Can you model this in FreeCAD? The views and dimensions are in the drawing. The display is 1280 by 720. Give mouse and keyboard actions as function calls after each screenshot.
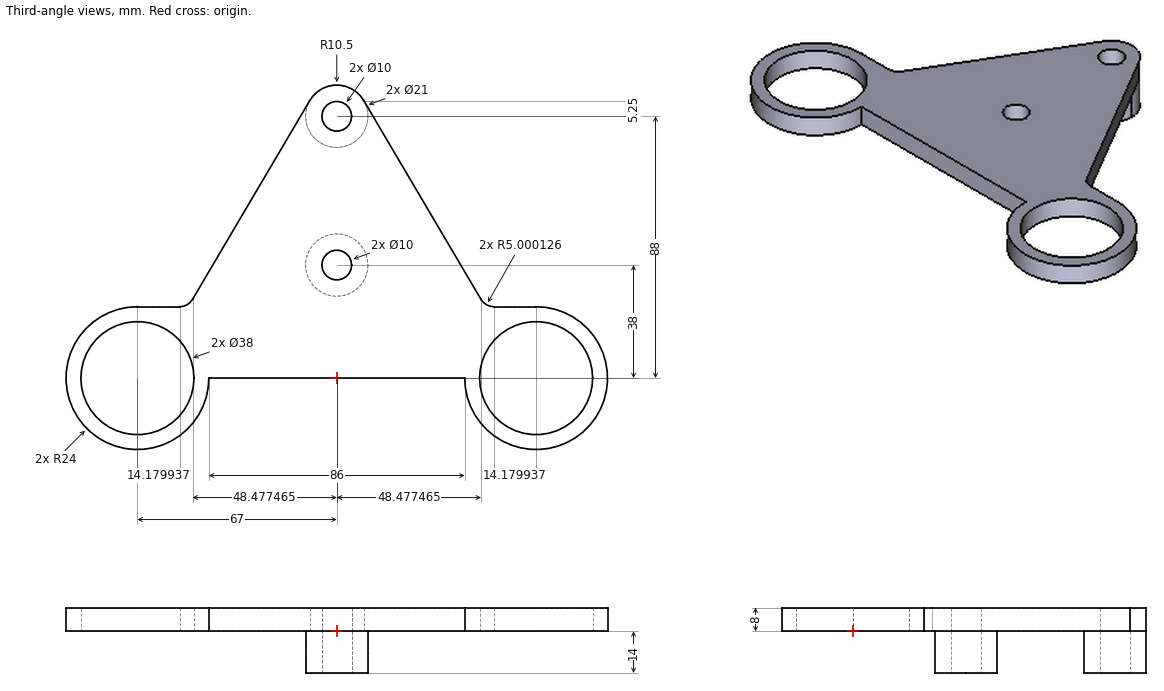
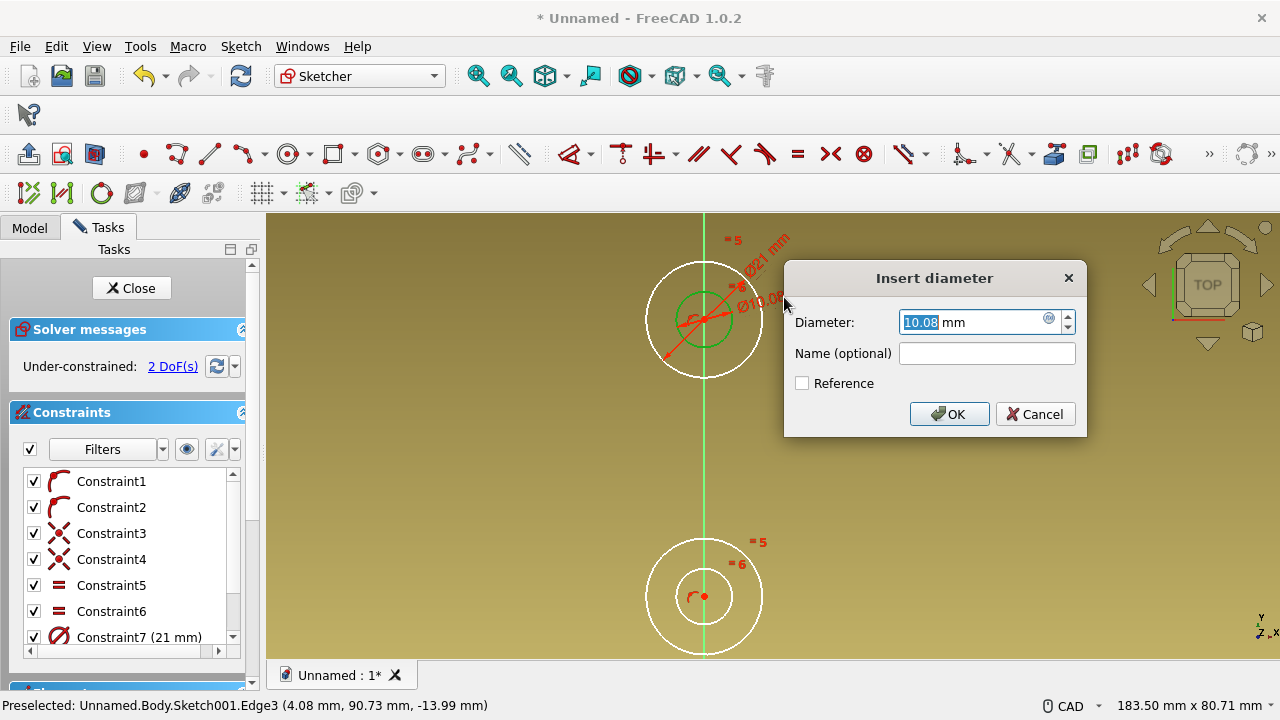
text(10)
key(Return)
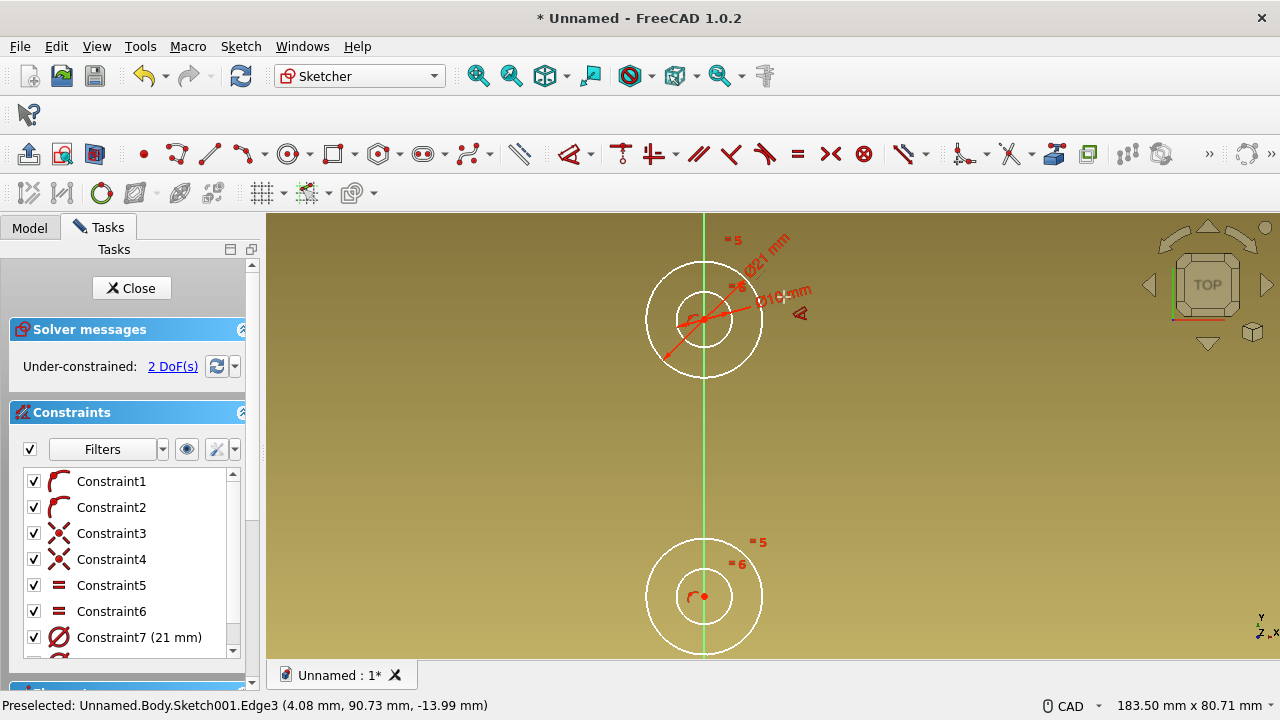
click(704, 320)
click(738, 475)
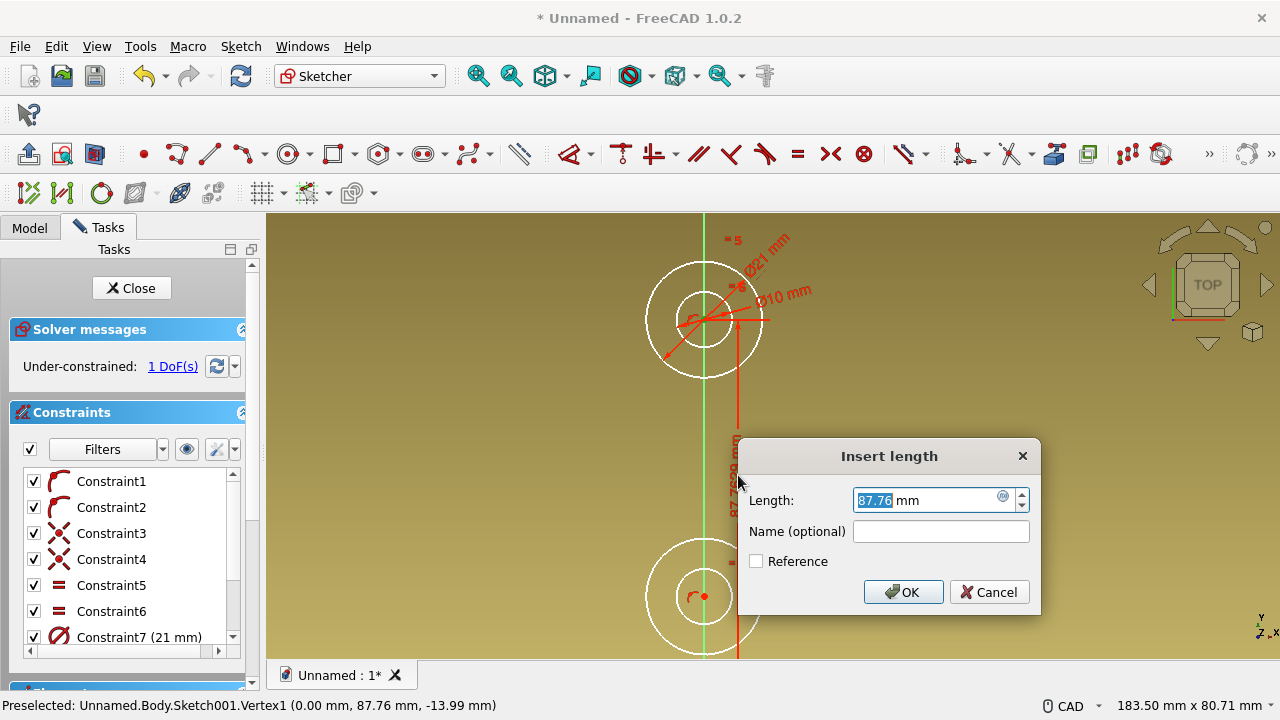
text(88)
key(Return)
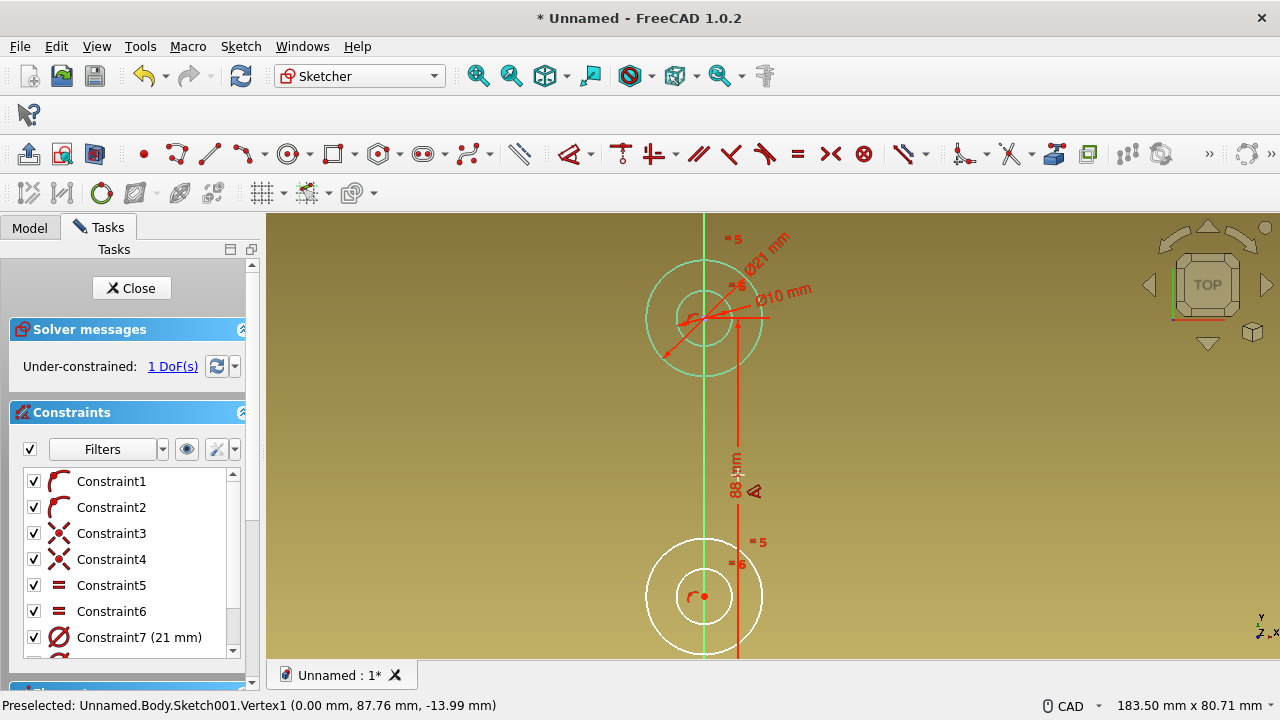
click(704, 597)
click(738, 622)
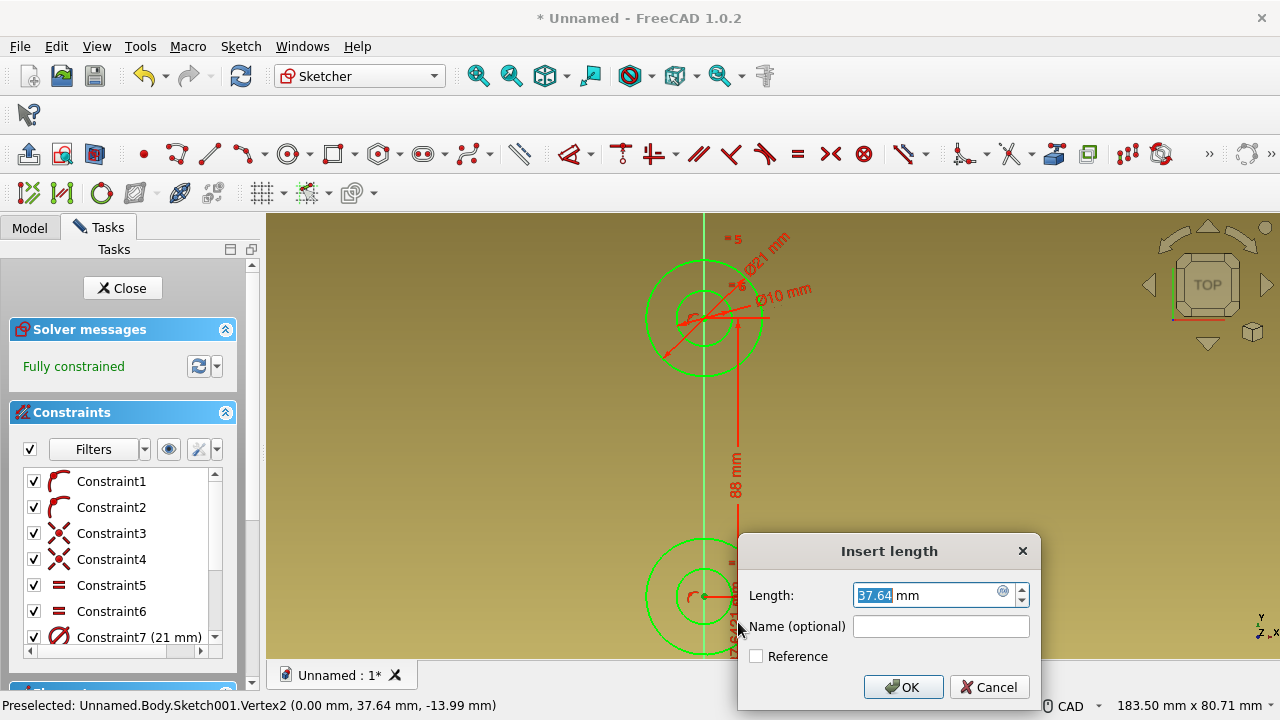
text(38)
key(Return)
key(Escape)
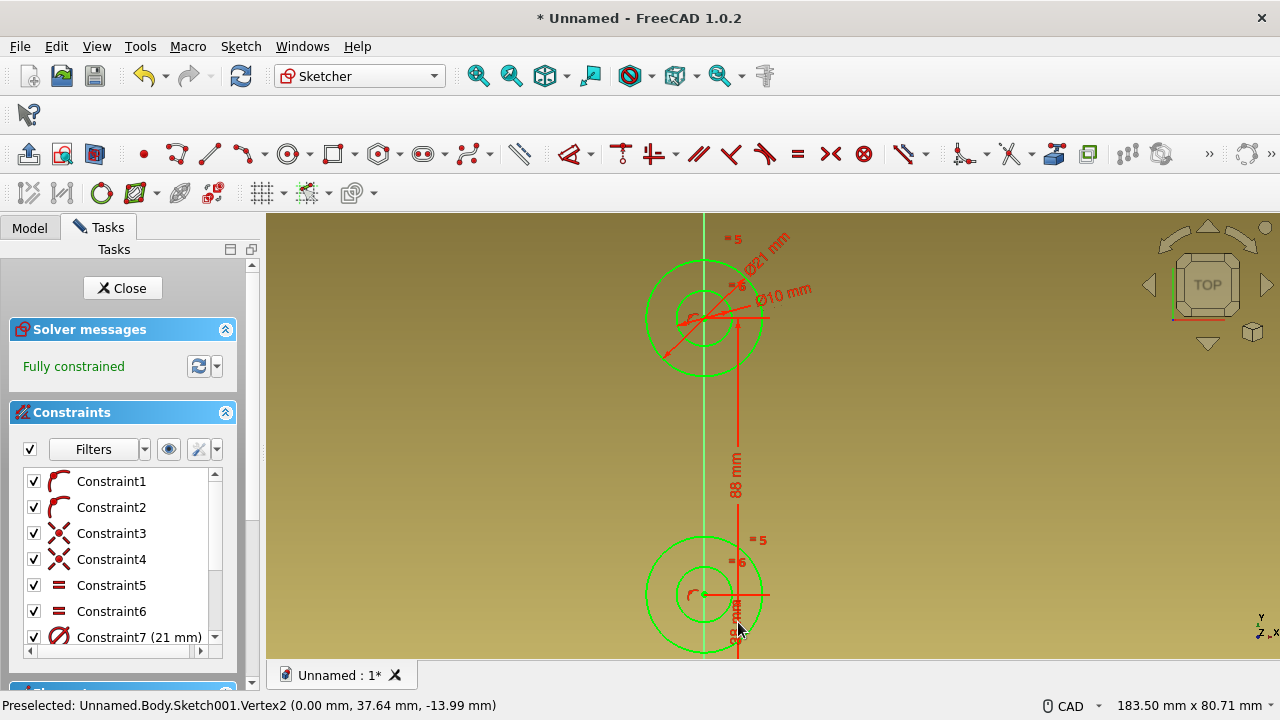
click(123, 288)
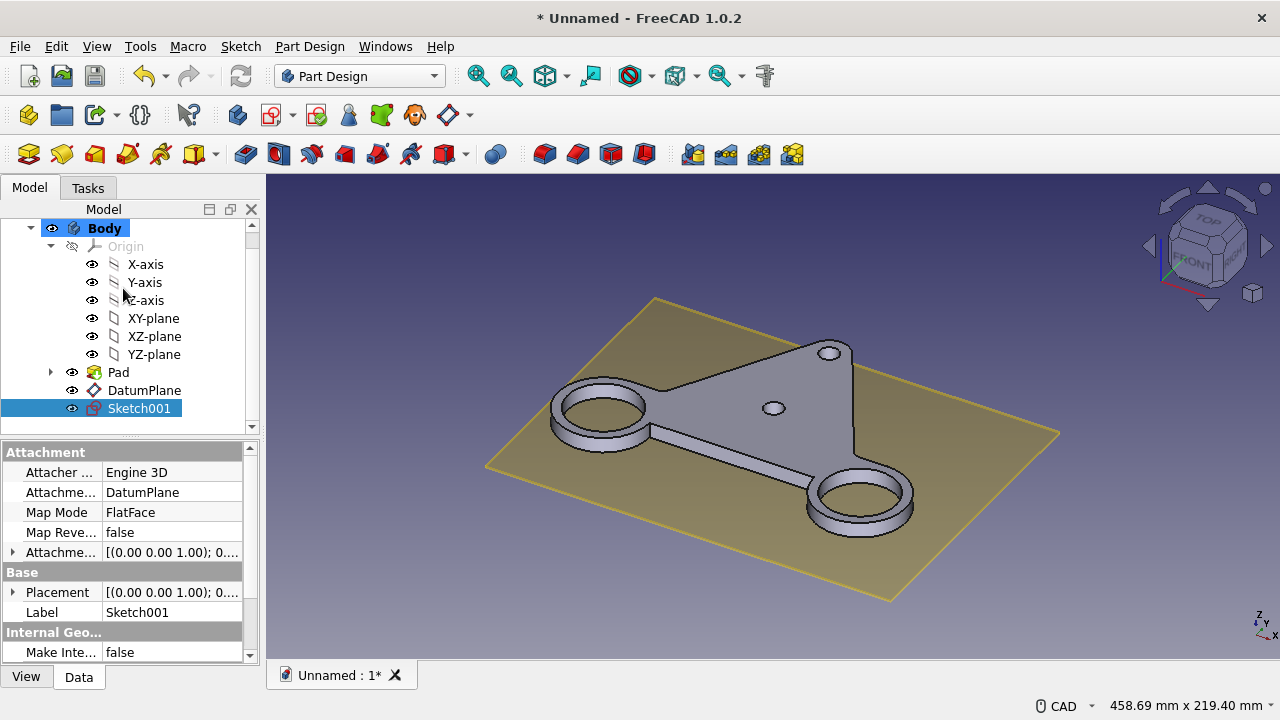
click(29, 154)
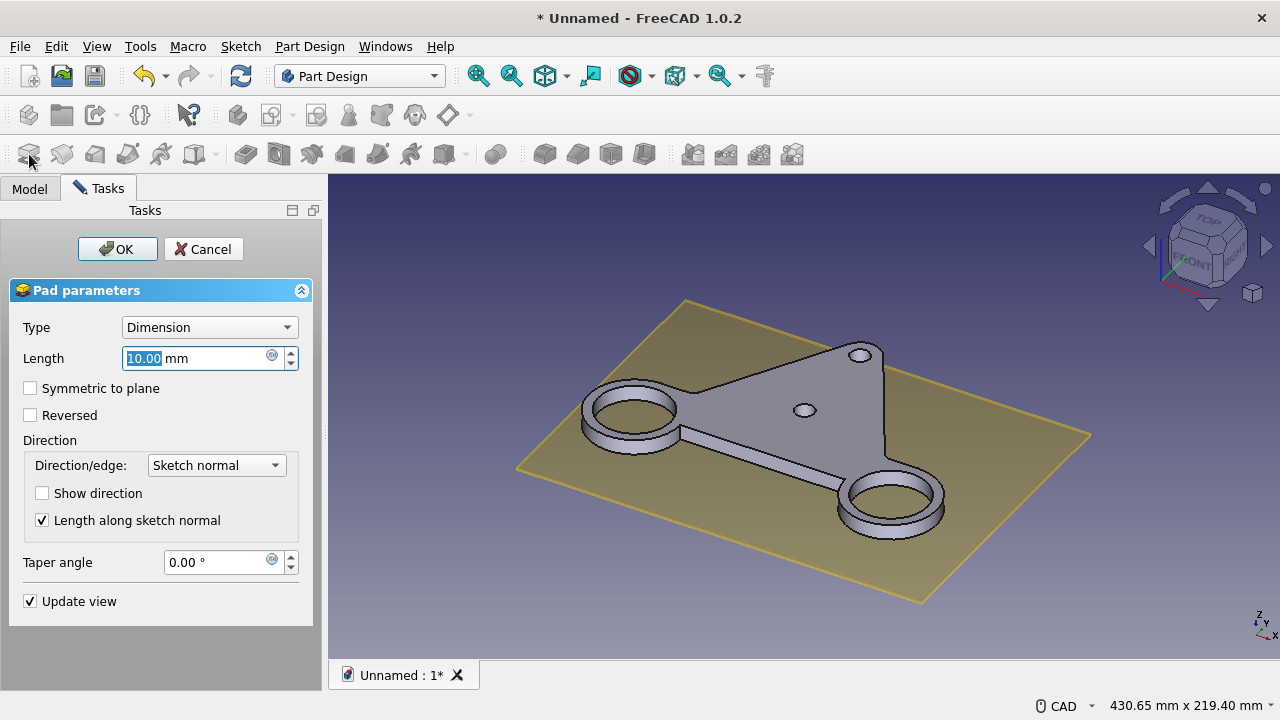
text(14)
key(Tab)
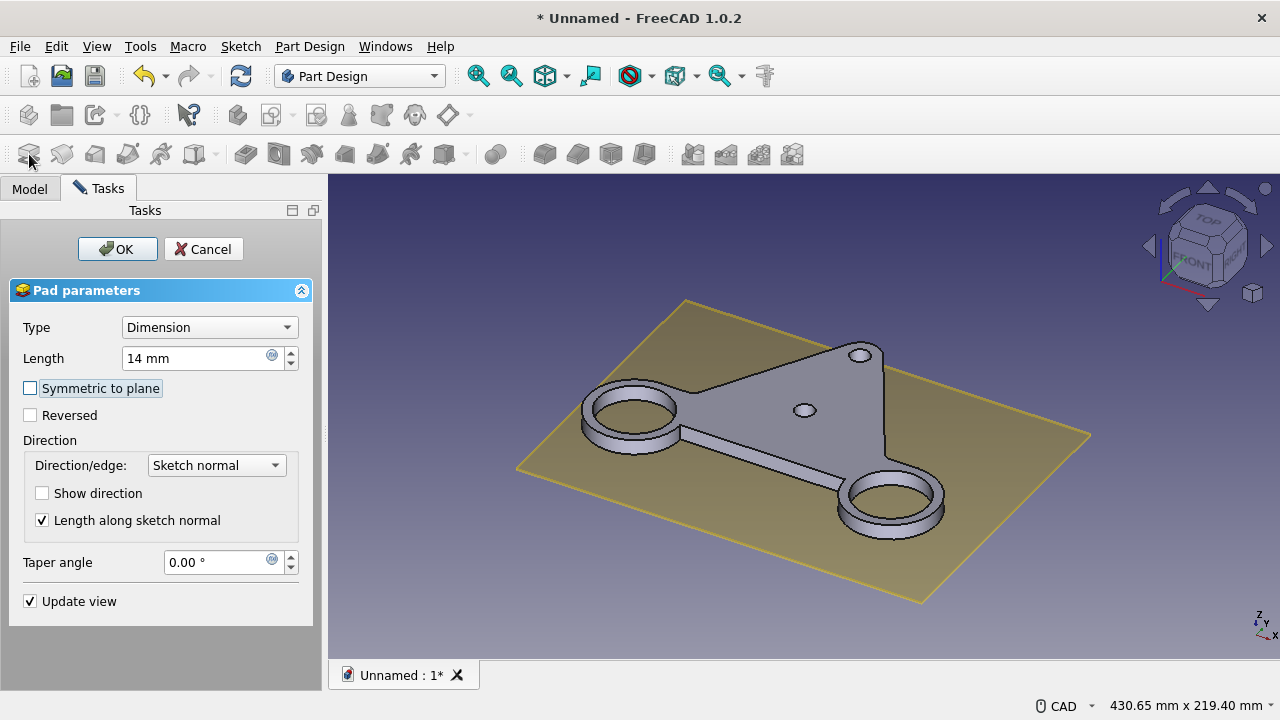
click(118, 249)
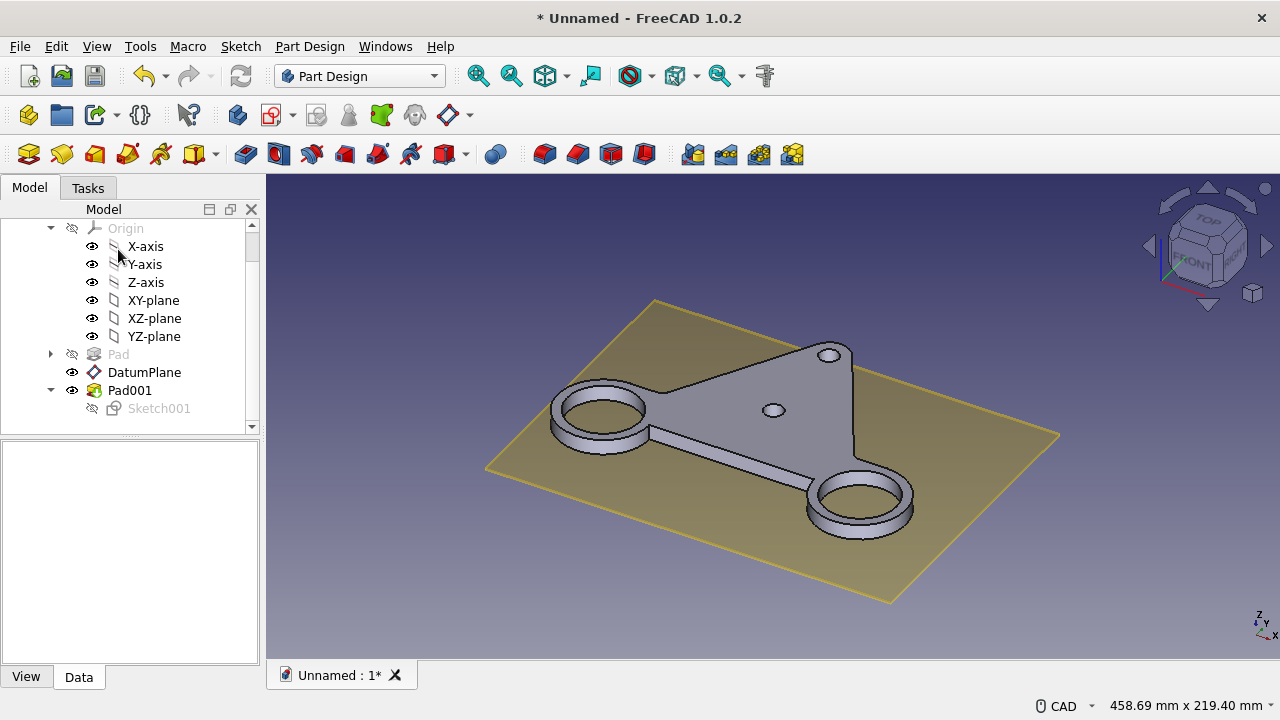
click(117, 372)
key(space)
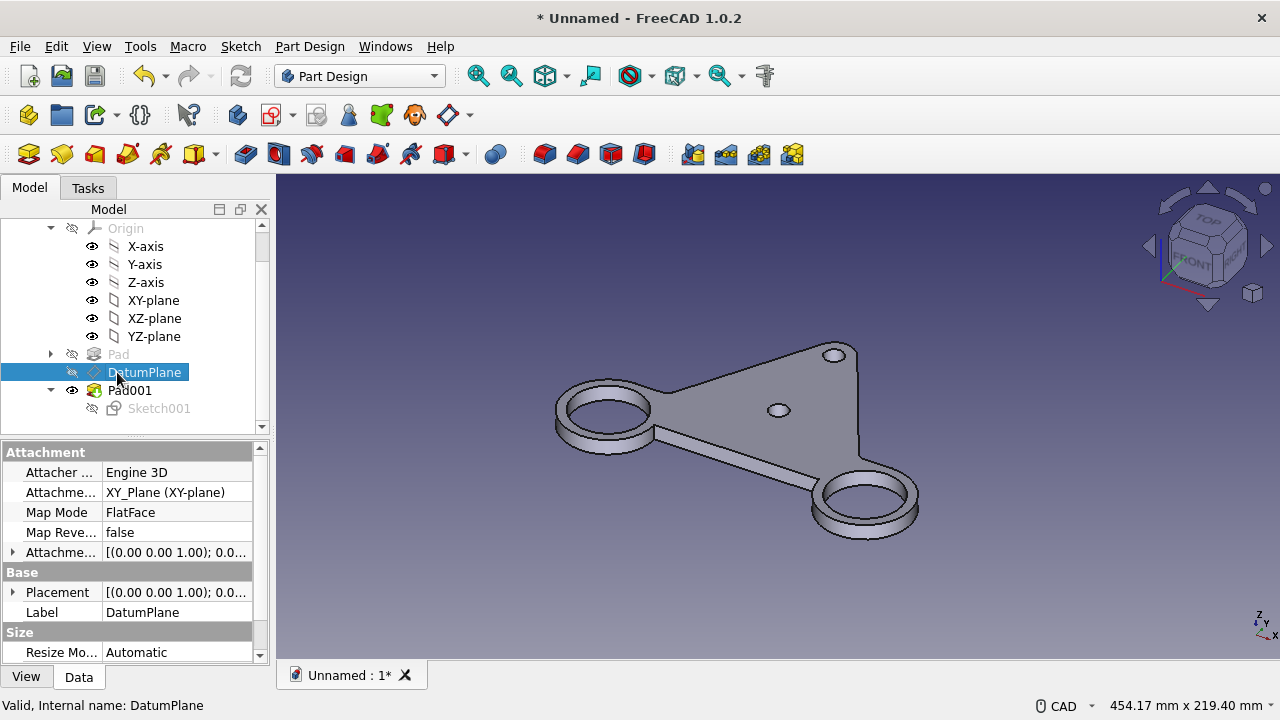
key(0)